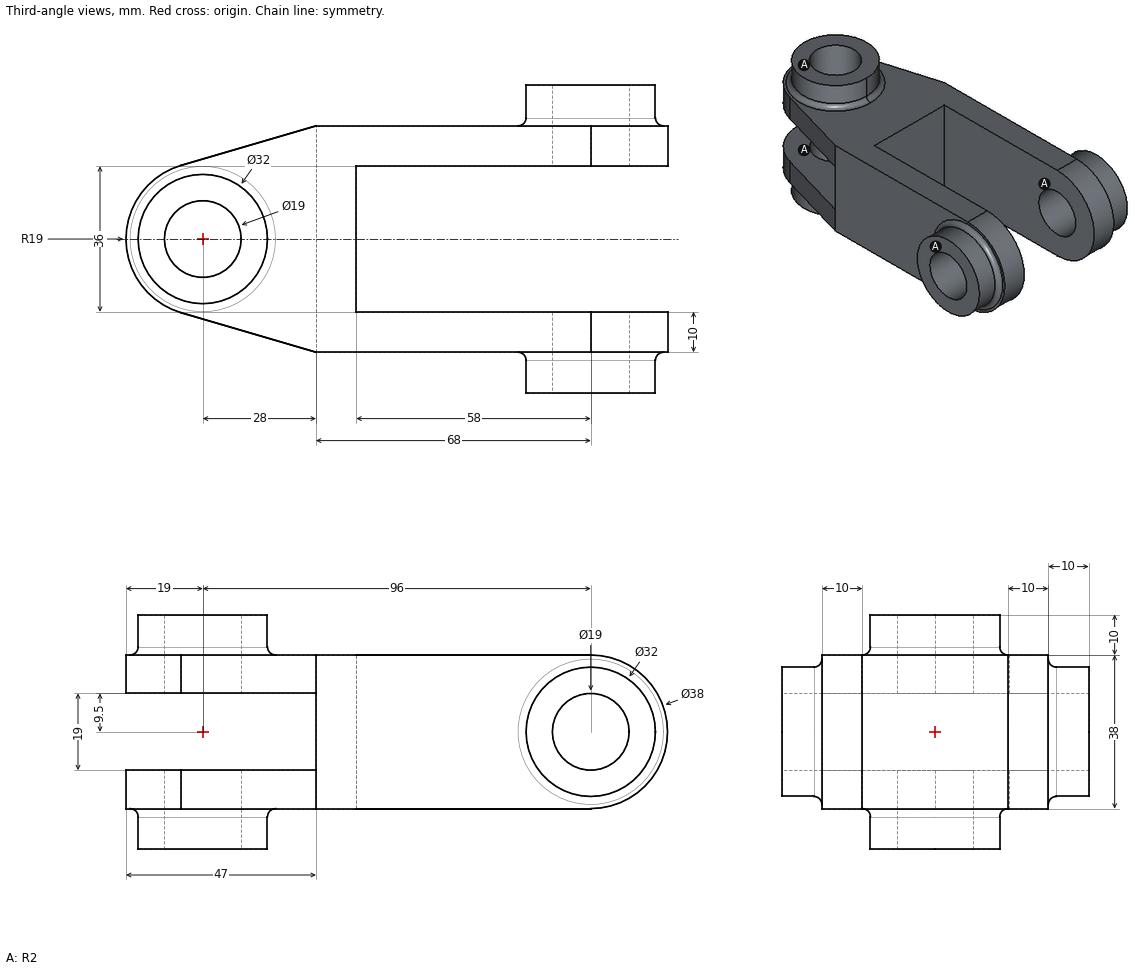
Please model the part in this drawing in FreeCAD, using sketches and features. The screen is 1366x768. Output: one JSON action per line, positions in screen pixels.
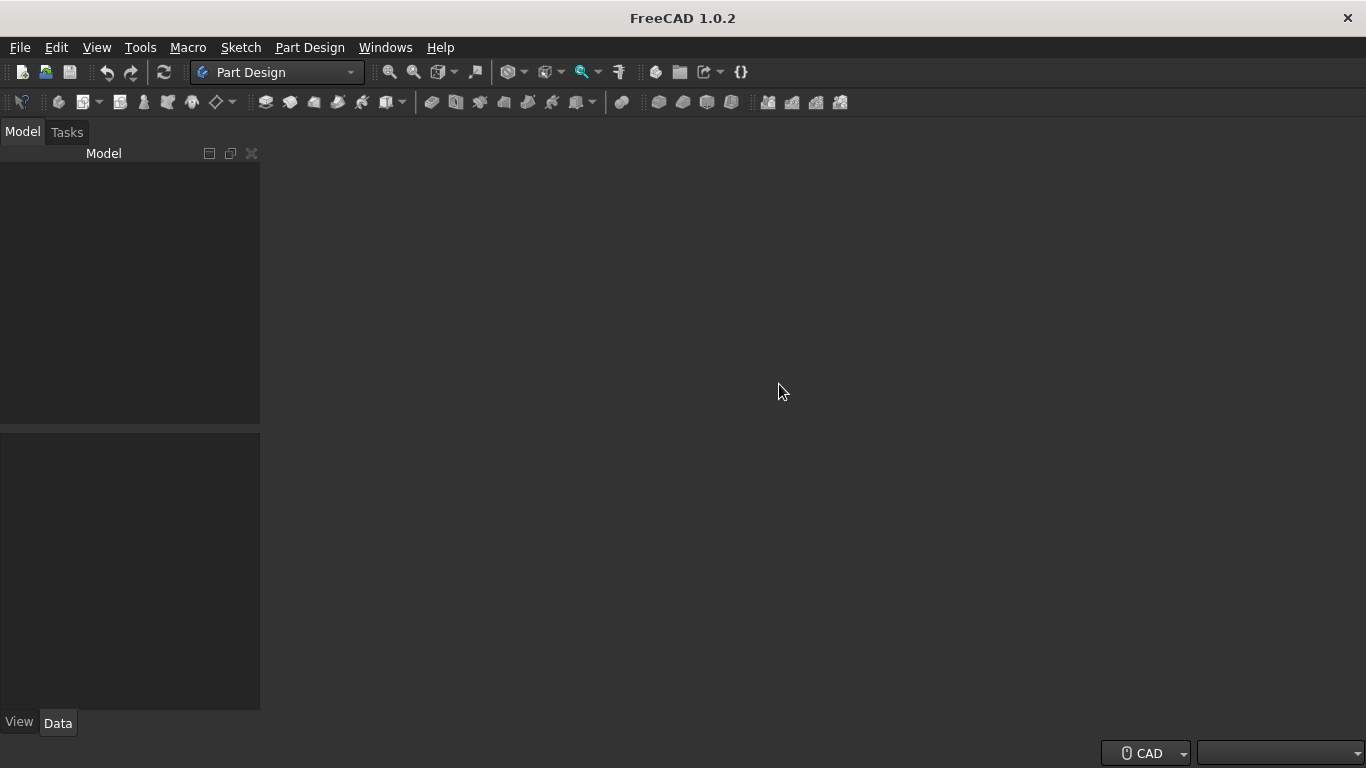
{"action": "key", "text": "ctrl+n"}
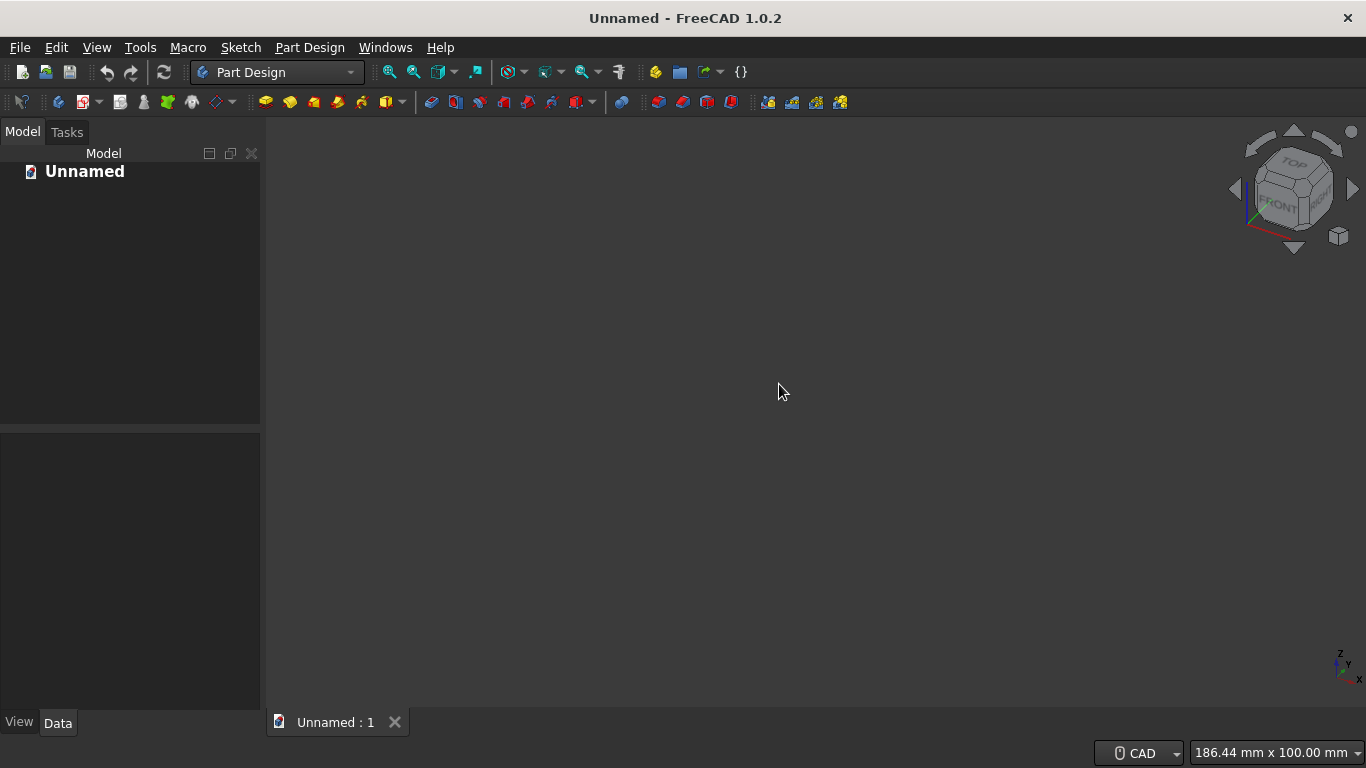
{"action": "left_click", "coordinate": [84, 102]}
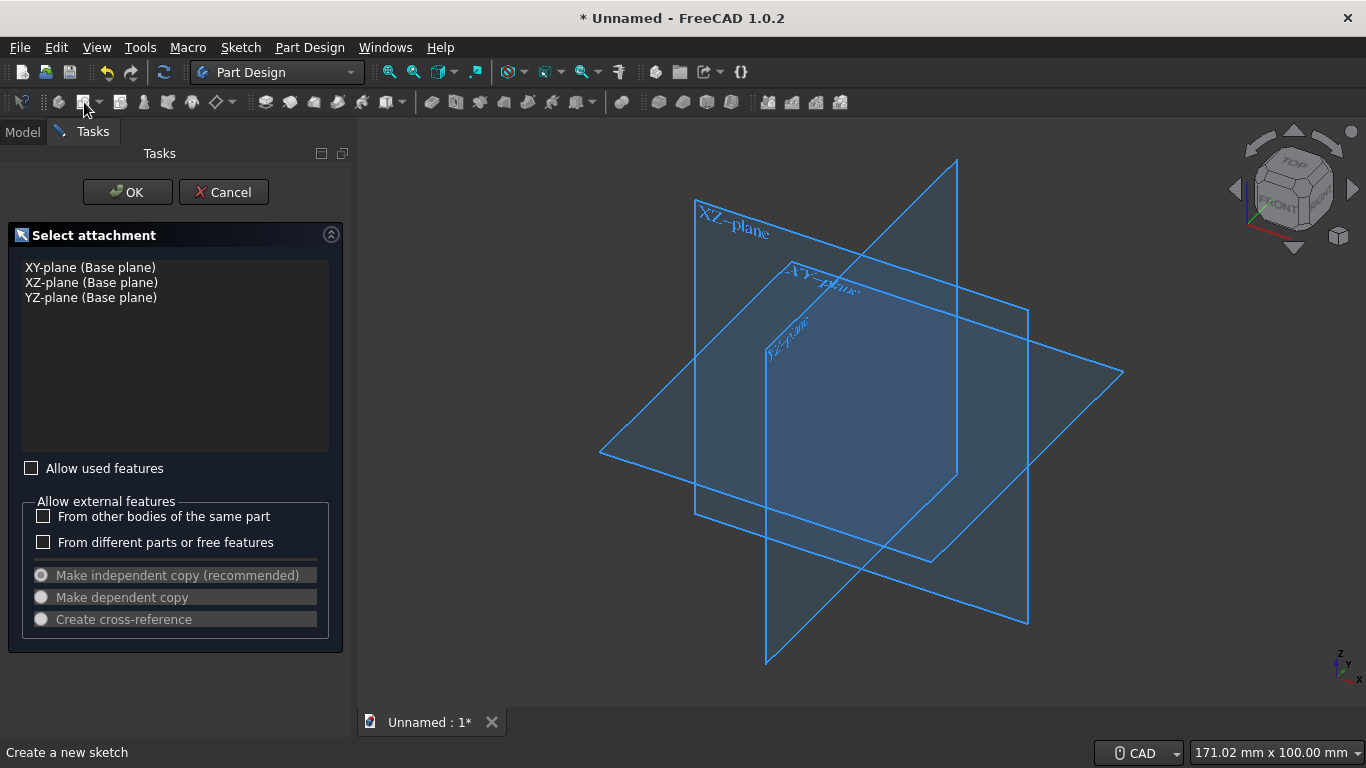
{"action": "left_click", "coordinate": [82, 268]}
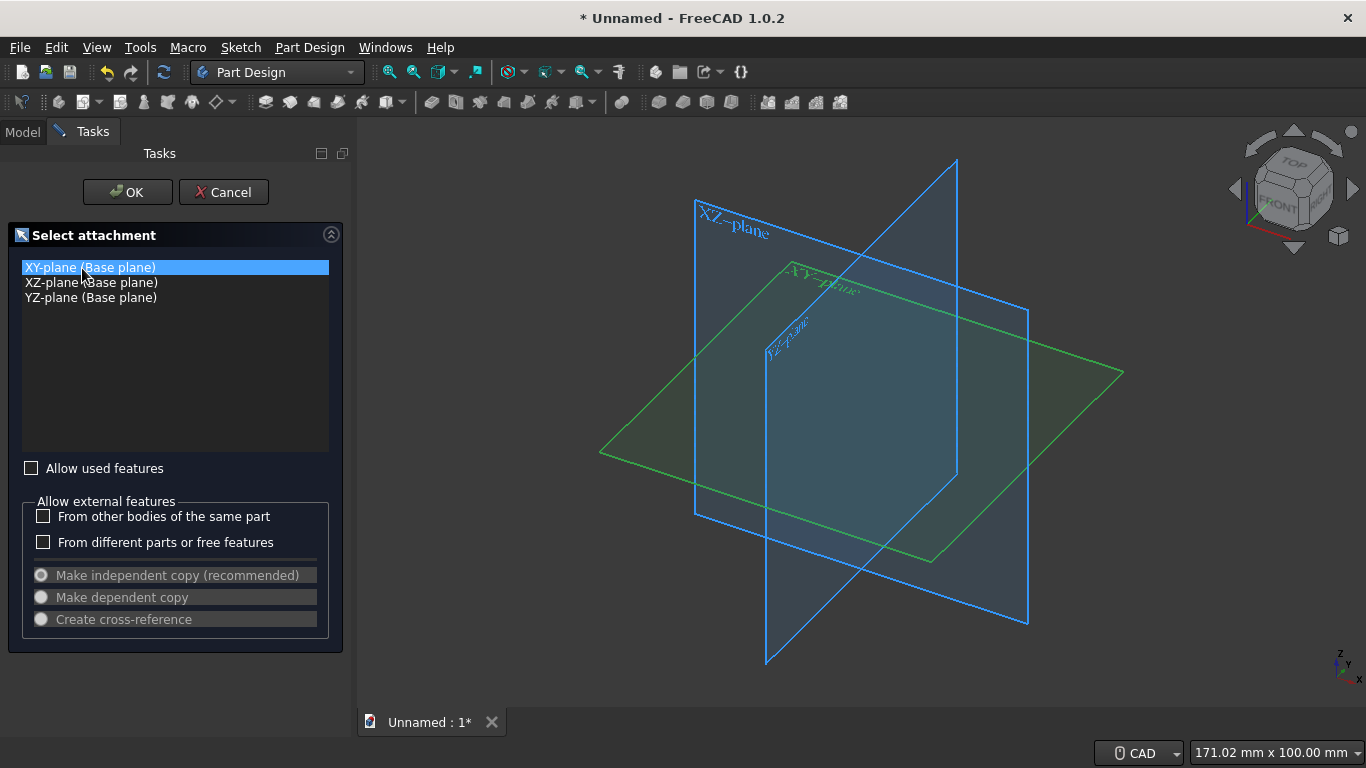
{"action": "left_click", "coordinate": [128, 192]}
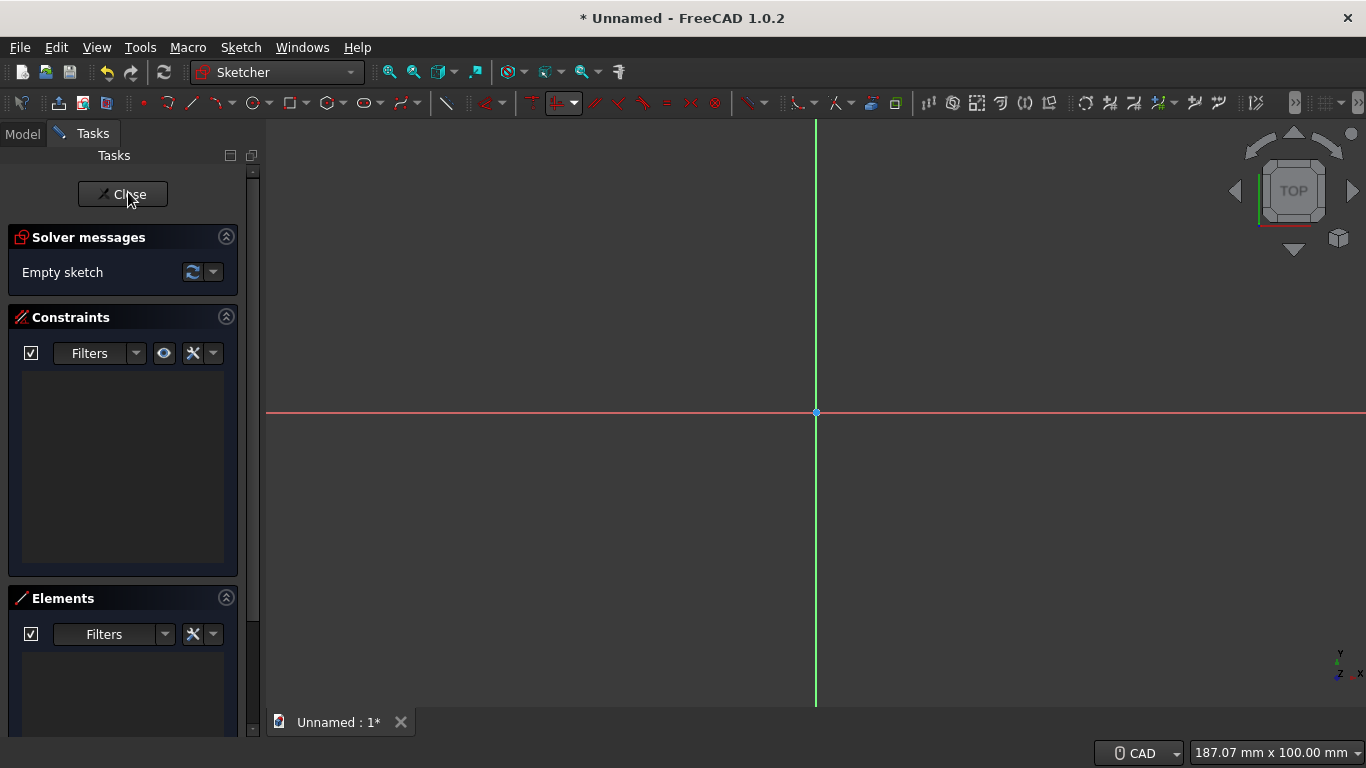
{"action": "scroll", "coordinate": [294, 413], "scroll_direction": "down", "scroll_amount": 2}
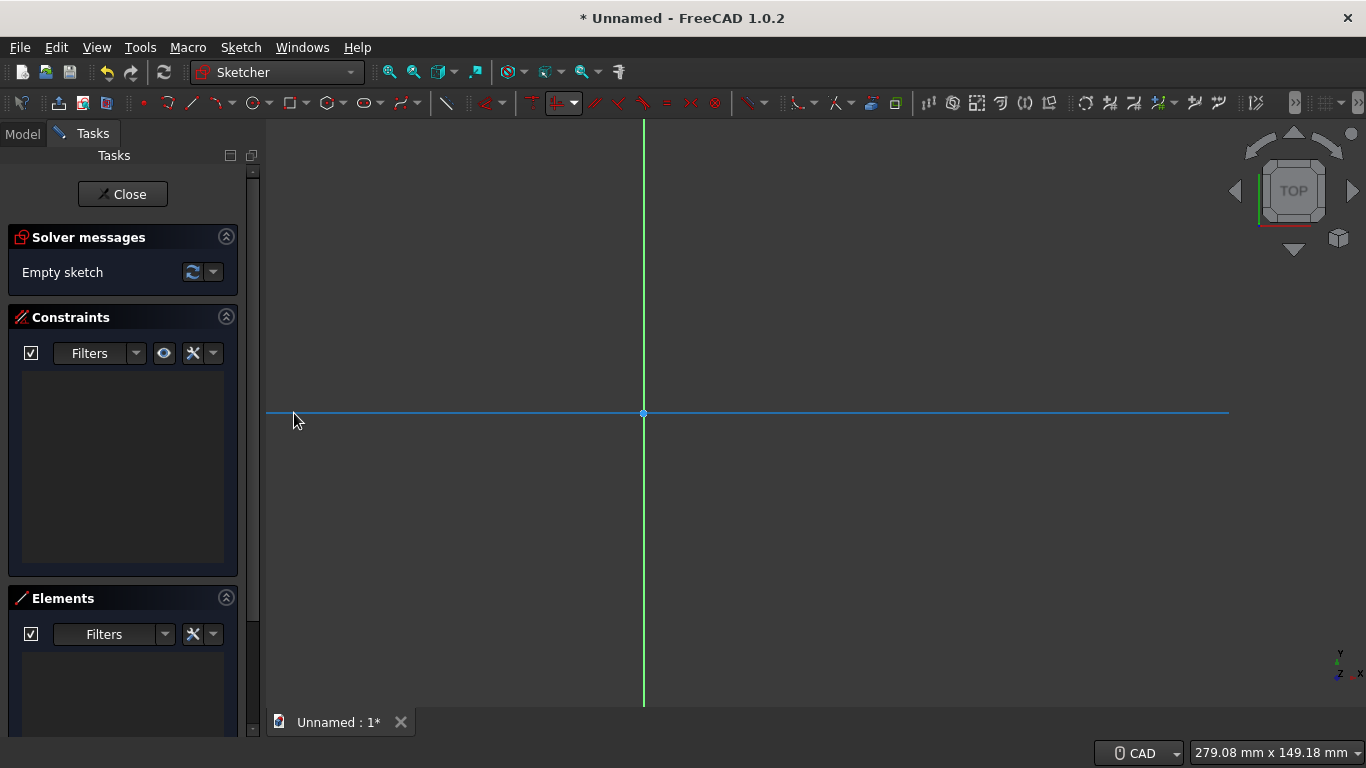
{"action": "scroll", "coordinate": [894, 414], "scroll_direction": "up", "scroll_amount": 2}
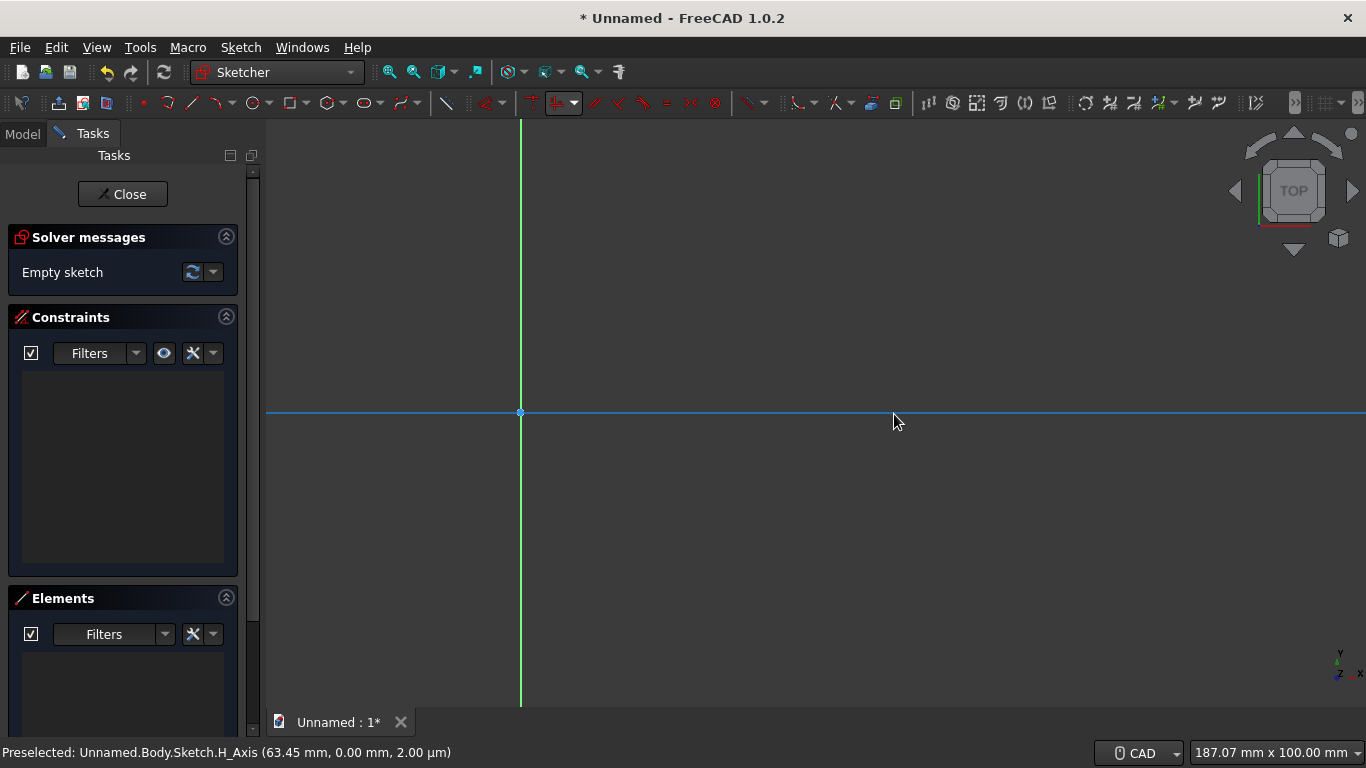
{"action": "left_click", "coordinate": [168, 104]}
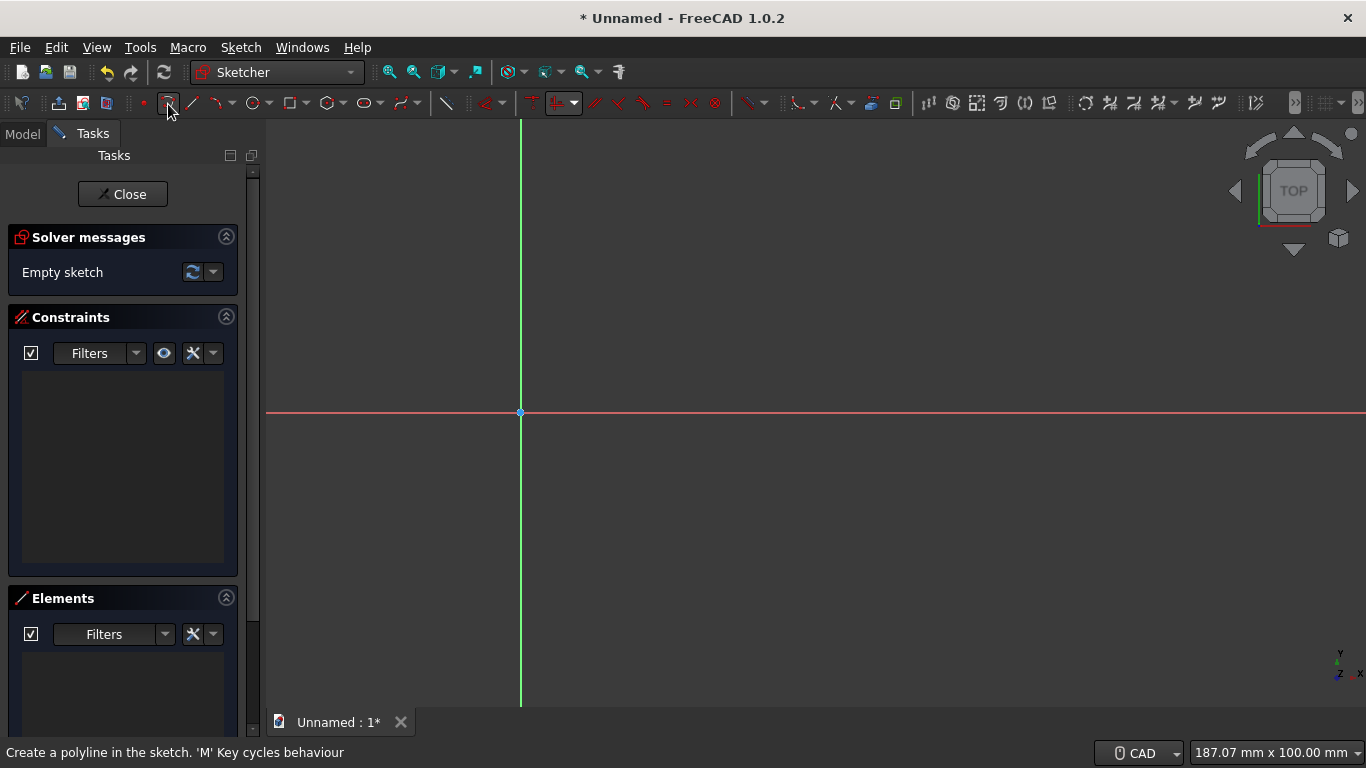
{"action": "left_click", "coordinate": [489, 520]}
{"action": "left_click", "coordinate": [685, 577]}
{"action": "left_click", "coordinate": [1085, 577]}
{"action": "left_click", "coordinate": [1085, 518]}
{"action": "left_click", "coordinate": [744, 518]}
{"action": "left_click", "coordinate": [744, 307]}
{"action": "left_click", "coordinate": [1085, 307]}
{"action": "left_click", "coordinate": [1085, 248]}
{"action": "left_click", "coordinate": [685, 248]}
{"action": "left_click", "coordinate": [489, 305]}
{"action": "right_click", "coordinate": [489, 305]}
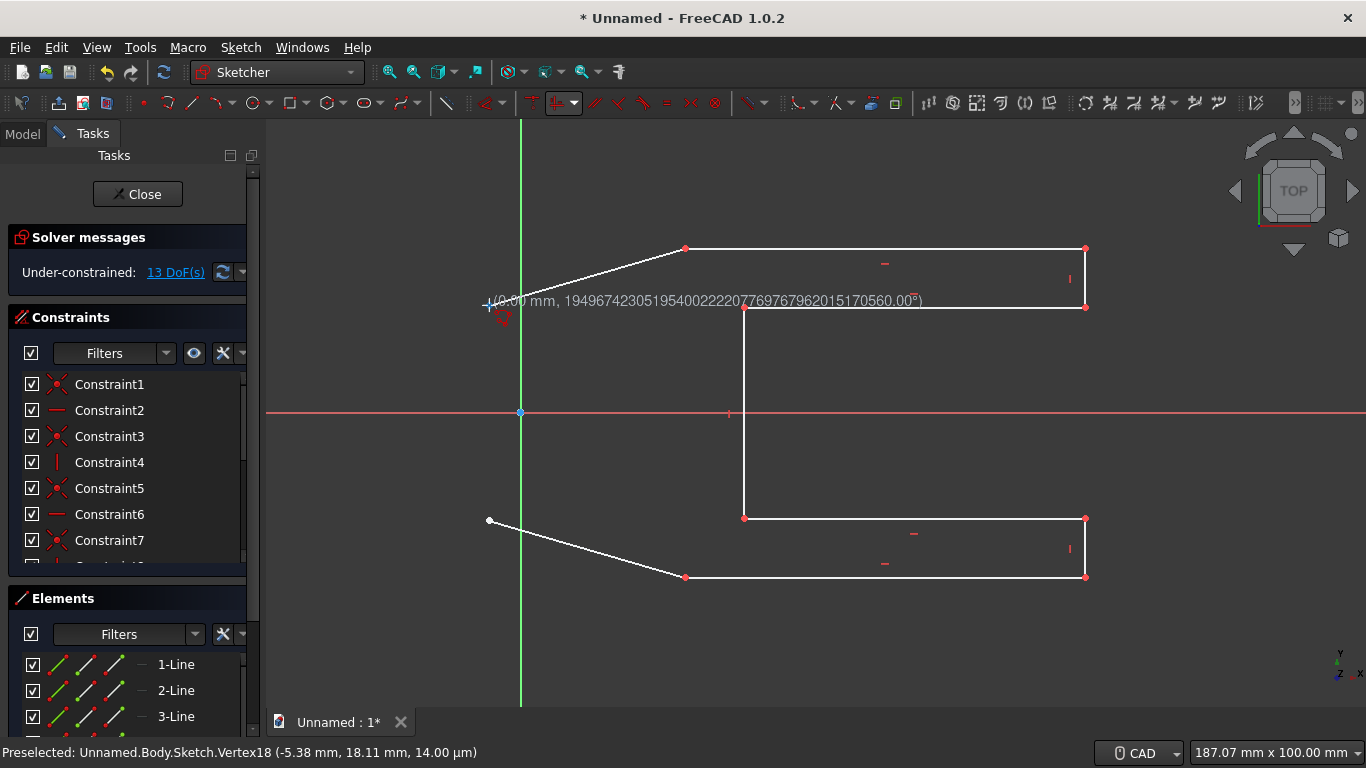
{"action": "left_click", "coordinate": [216, 104]}